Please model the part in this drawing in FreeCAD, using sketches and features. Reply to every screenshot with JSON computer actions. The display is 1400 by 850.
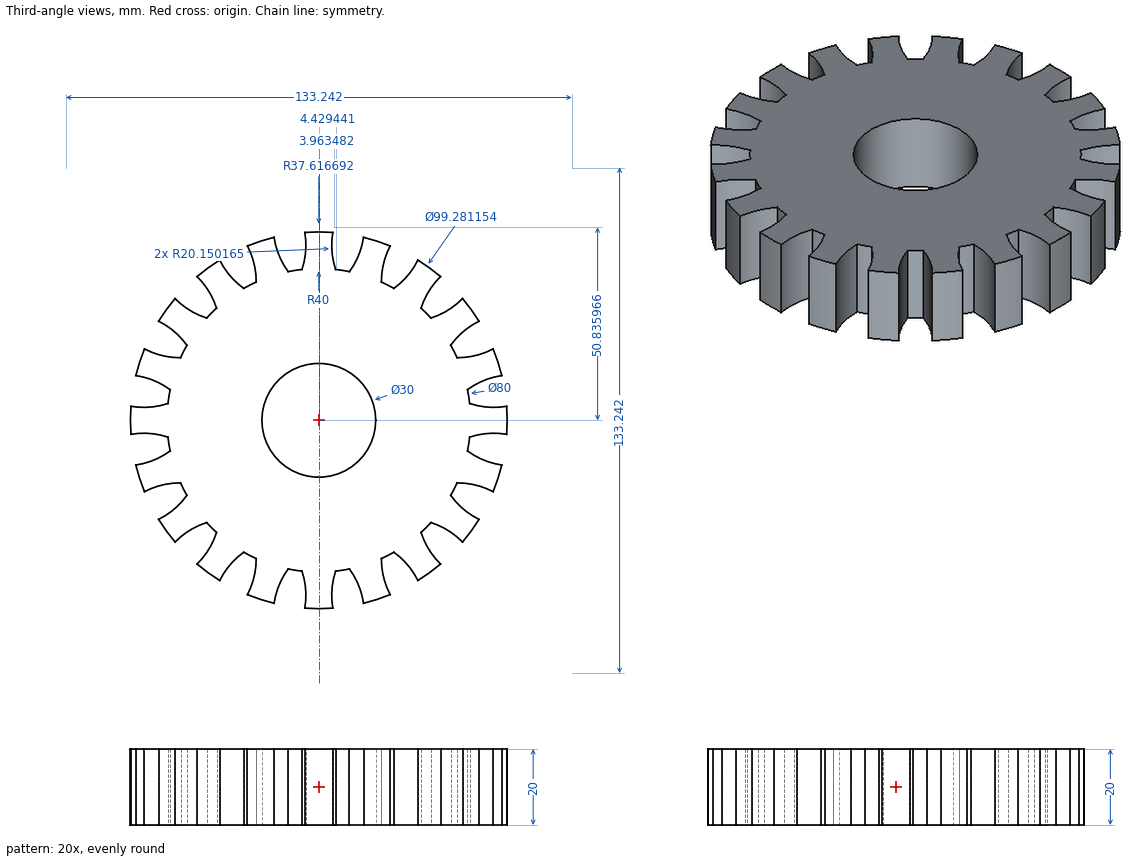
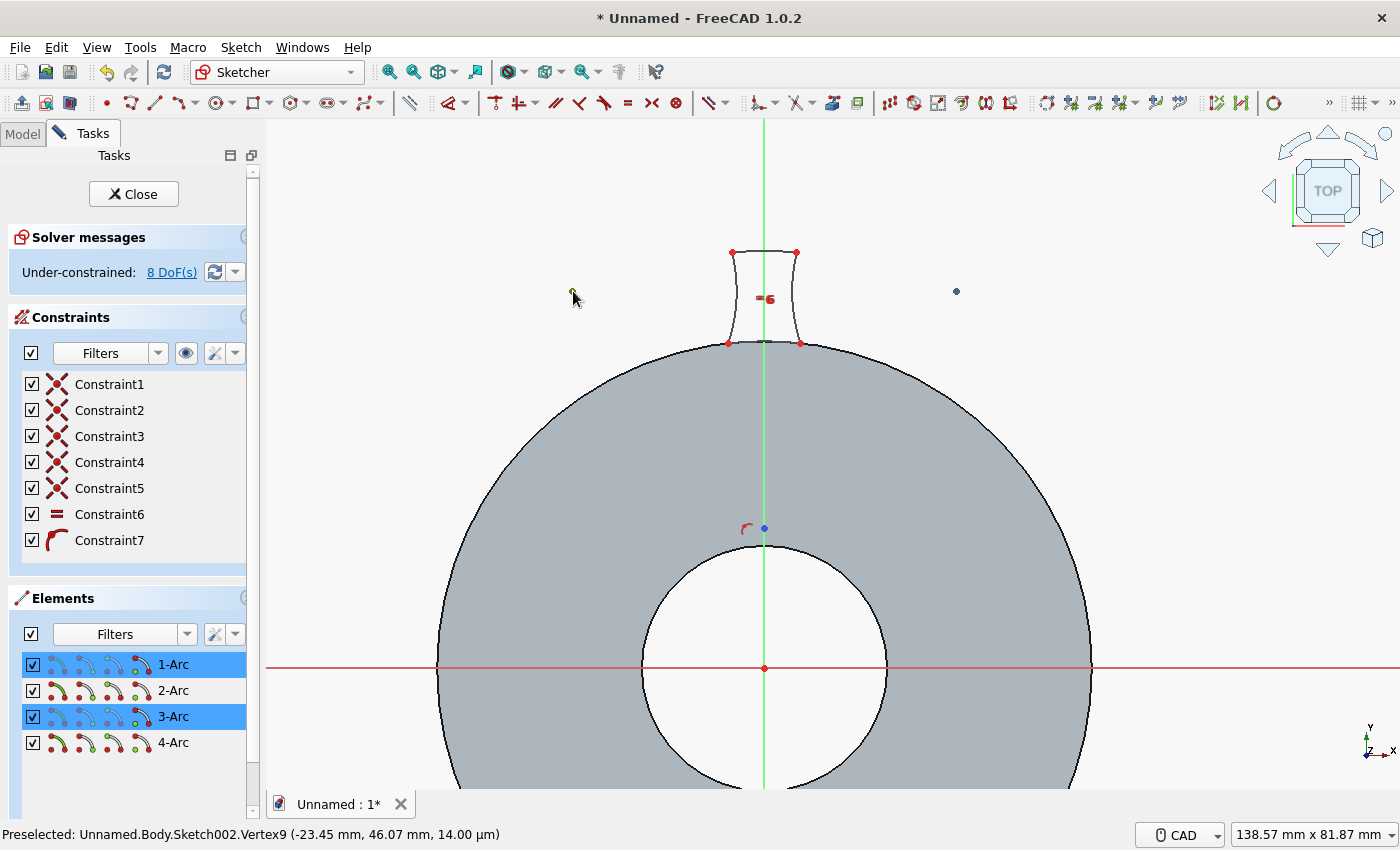
{"action": "left_click", "coordinate": [764, 717]}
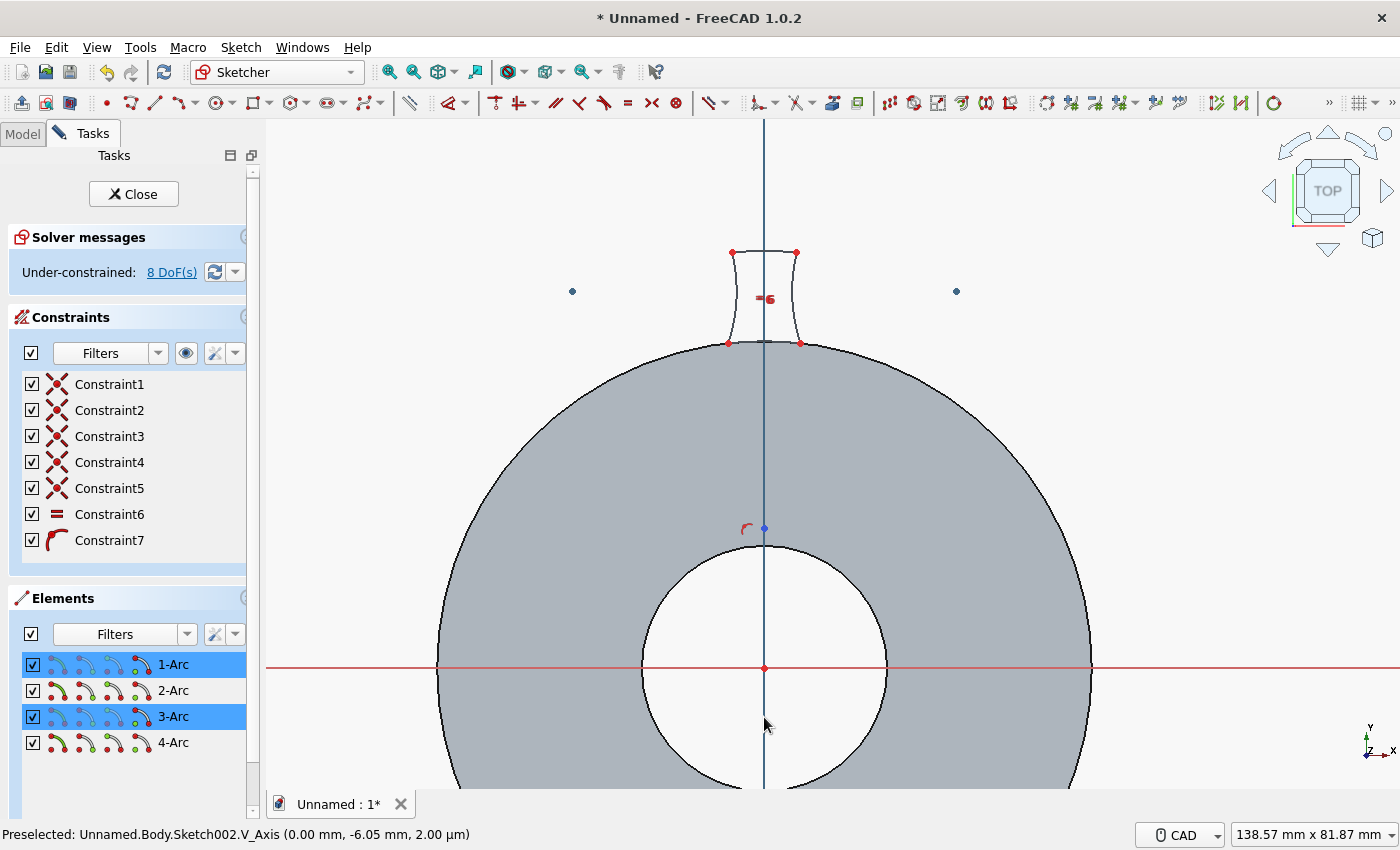
{"action": "left_click", "coordinate": [652, 104]}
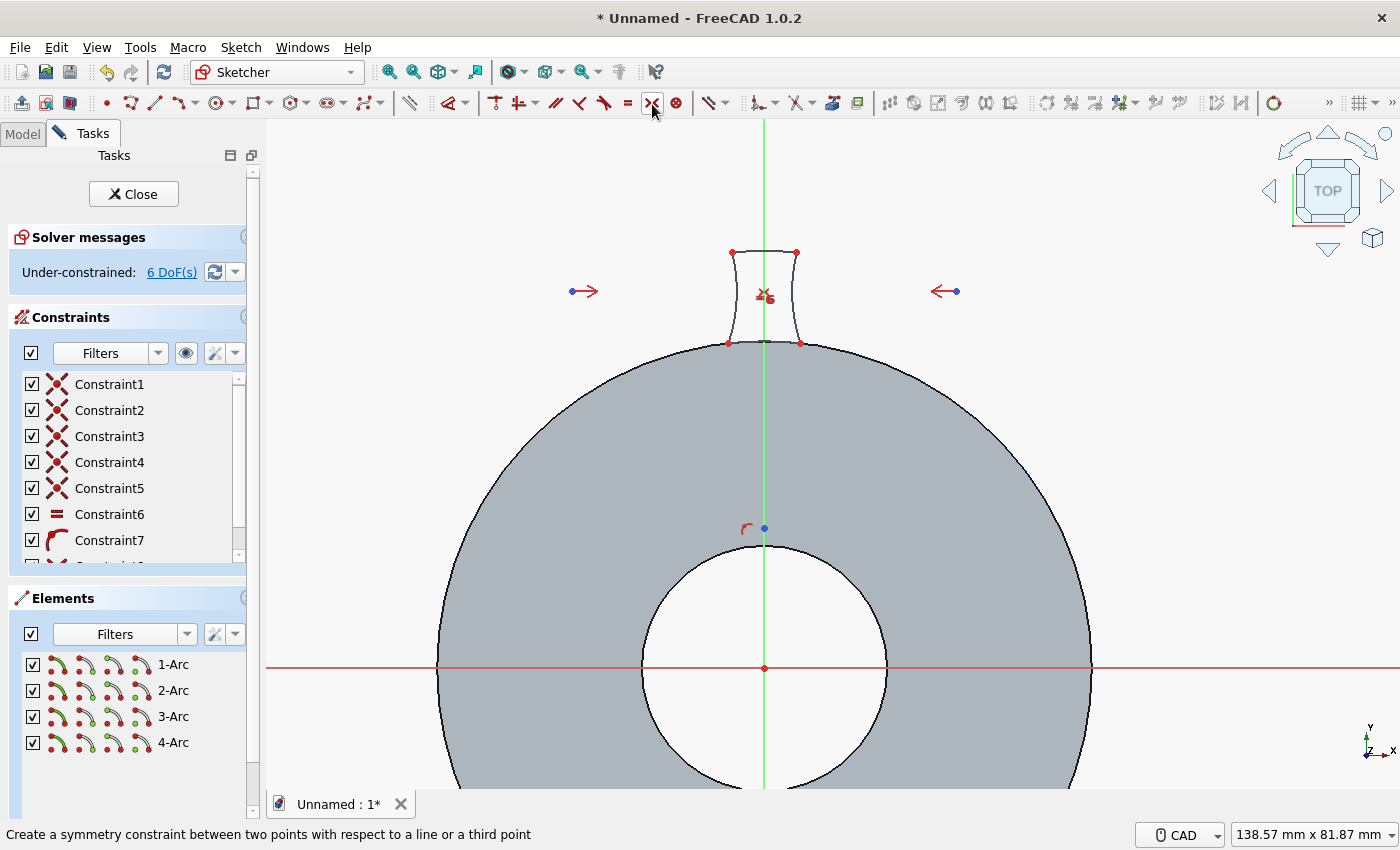
{"action": "left_click", "coordinate": [448, 104]}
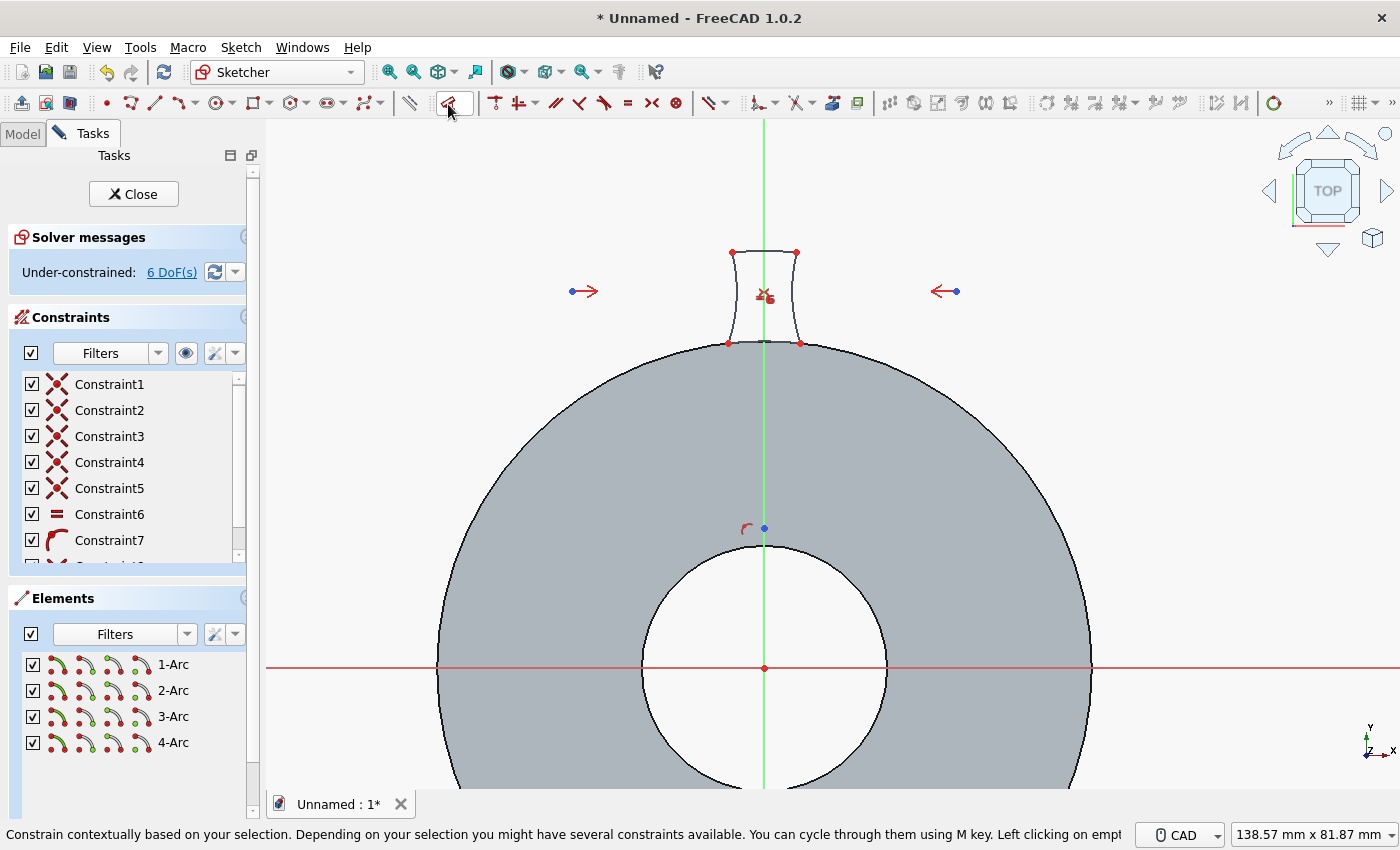
{"action": "left_click", "coordinate": [793, 280]}
{"action": "left_click", "coordinate": [792, 186]}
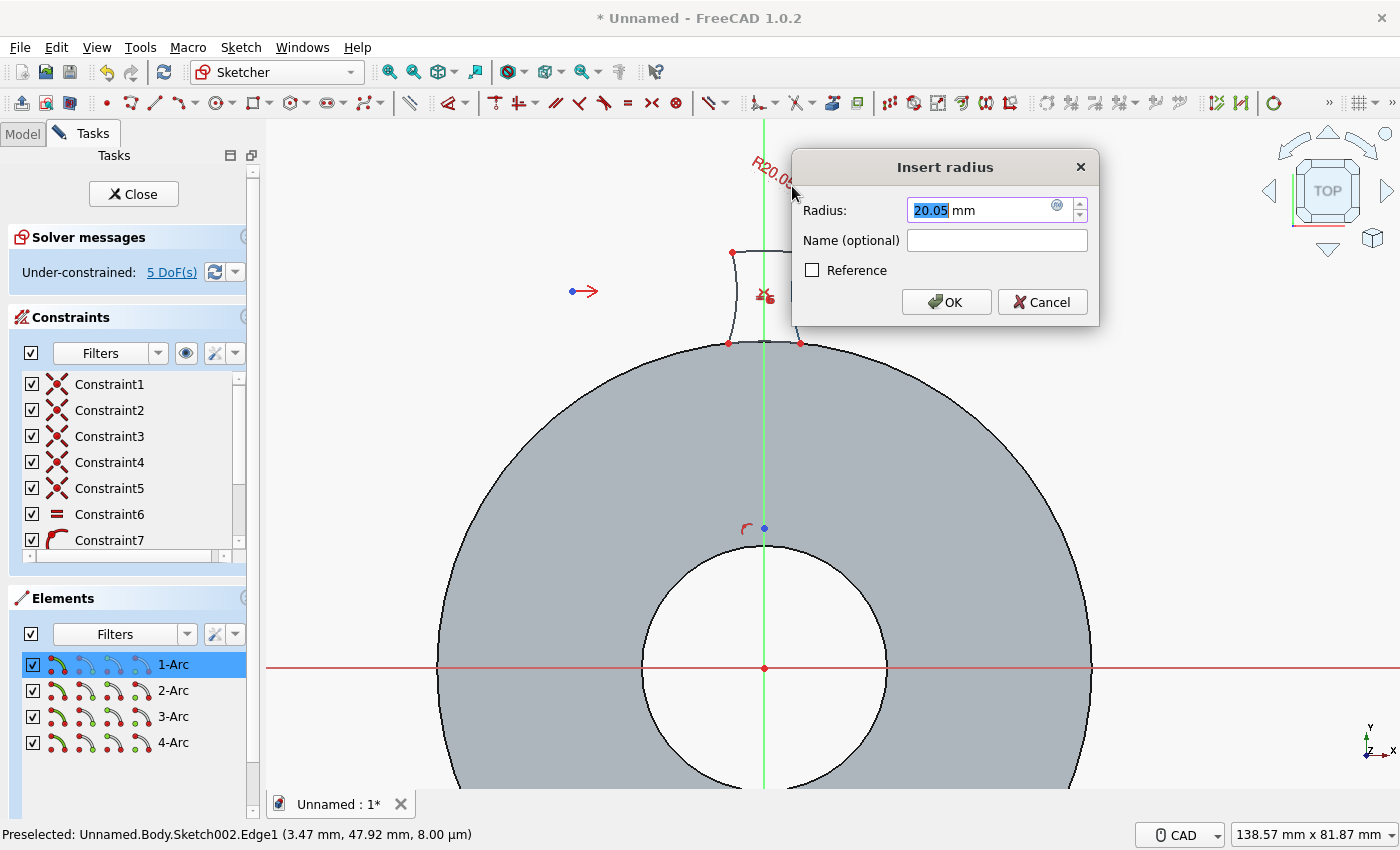
{"action": "type", "text": "20.150165"}
{"action": "key", "text": "Return"}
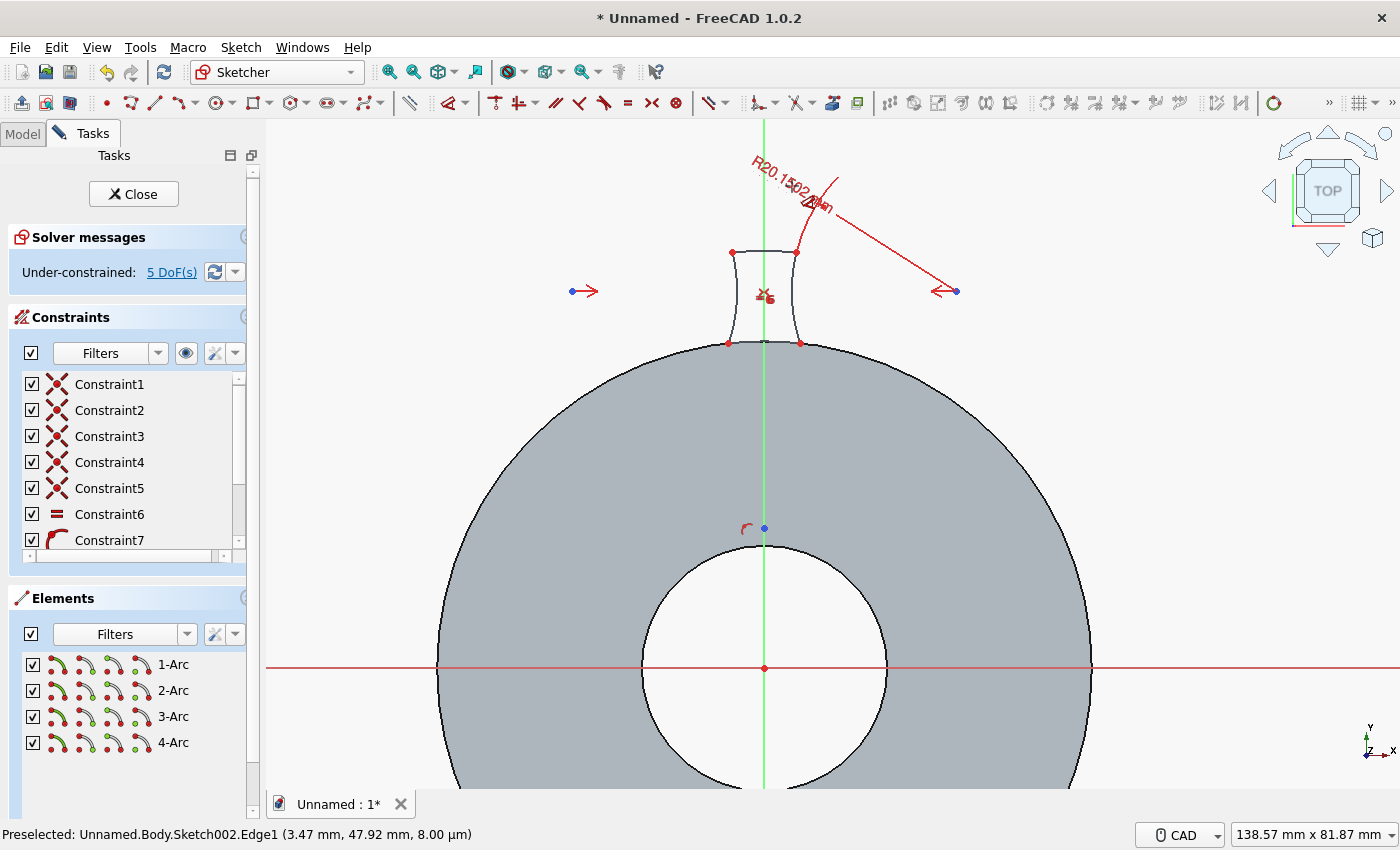
{"action": "left_click", "coordinate": [777, 251]}
{"action": "left_click", "coordinate": [778, 219]}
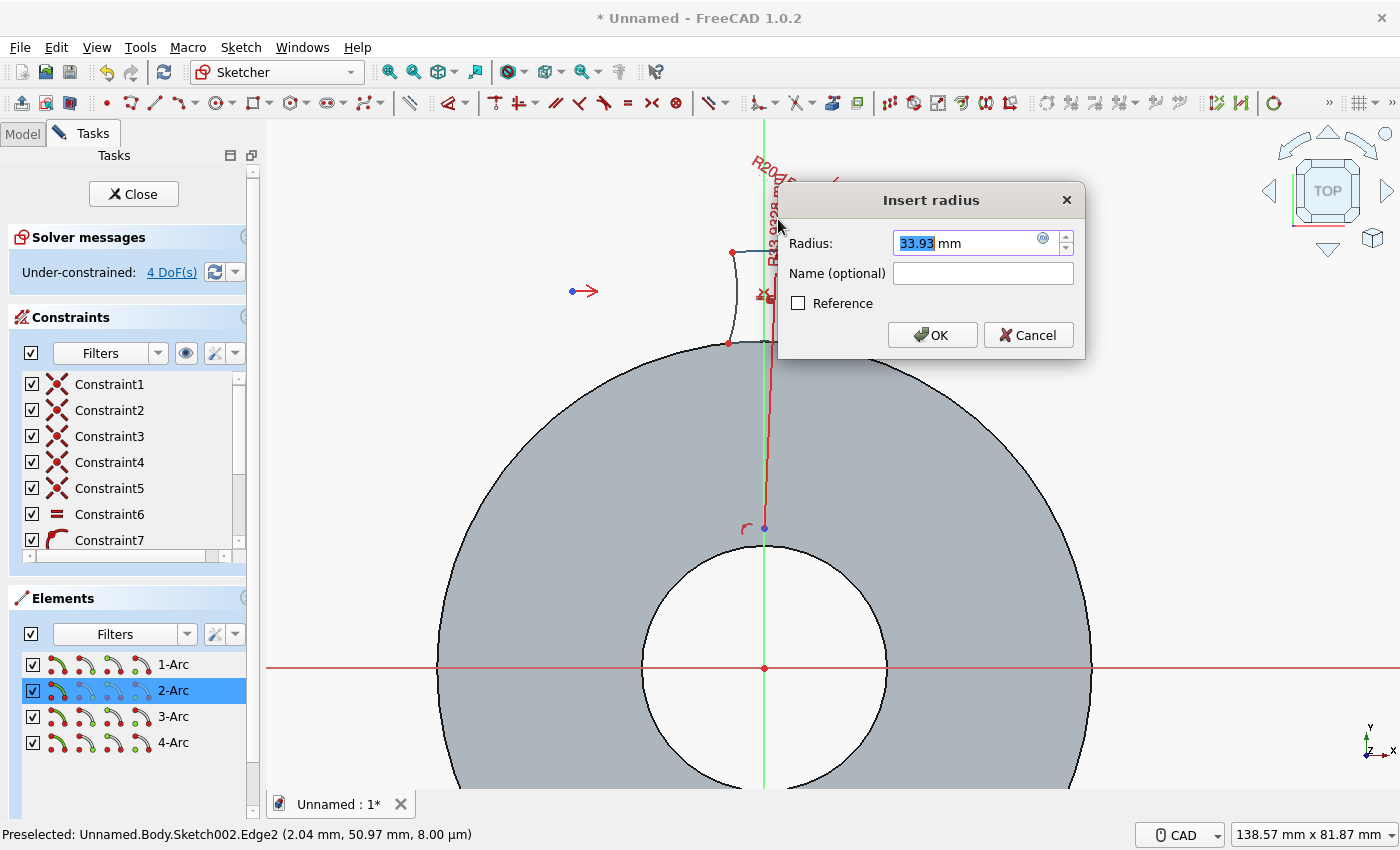
{"action": "type", "text": "37.616692"}
{"action": "key", "text": "Return"}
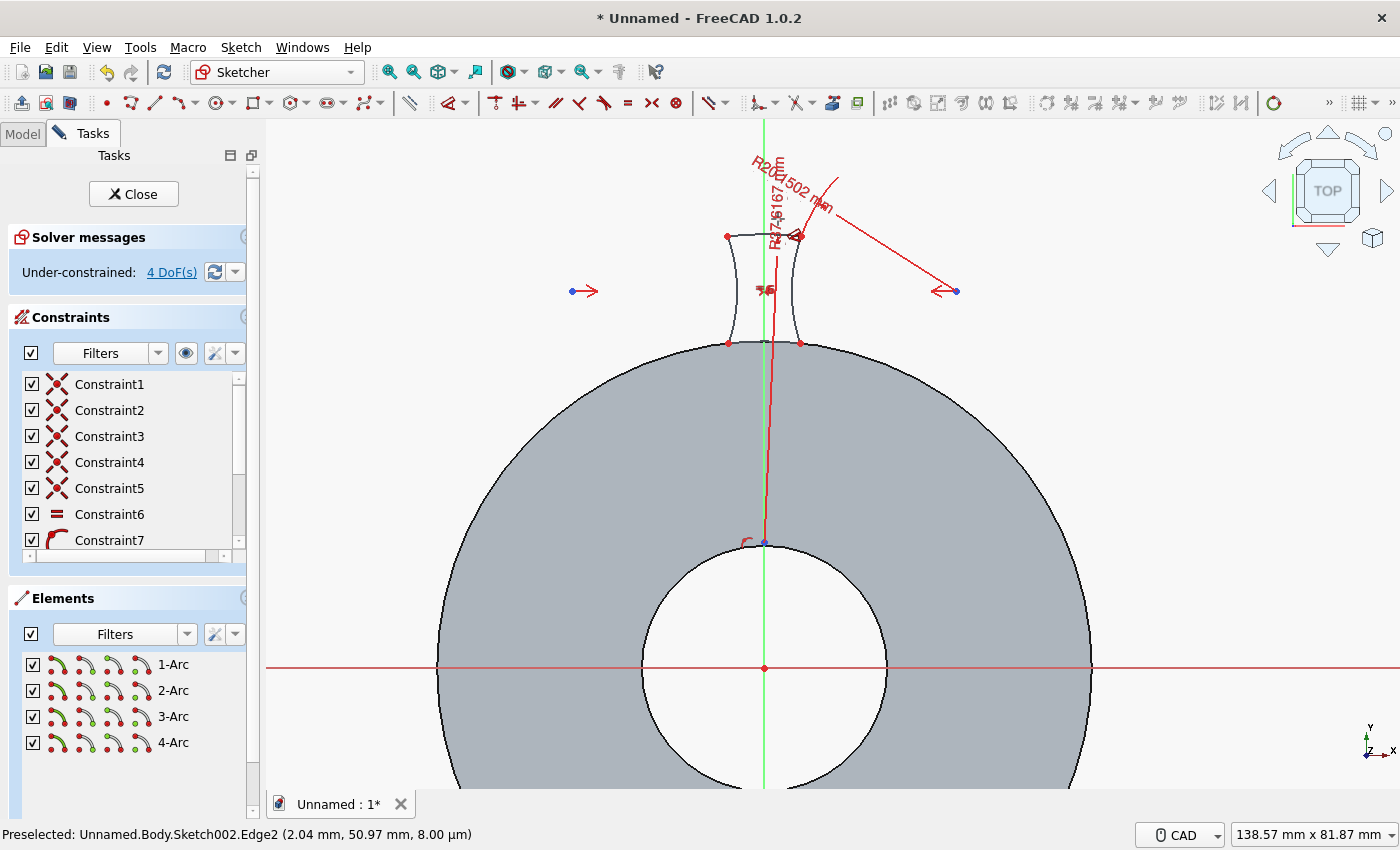
{"action": "left_click", "coordinate": [779, 342]}
{"action": "left_click", "coordinate": [950, 362]}